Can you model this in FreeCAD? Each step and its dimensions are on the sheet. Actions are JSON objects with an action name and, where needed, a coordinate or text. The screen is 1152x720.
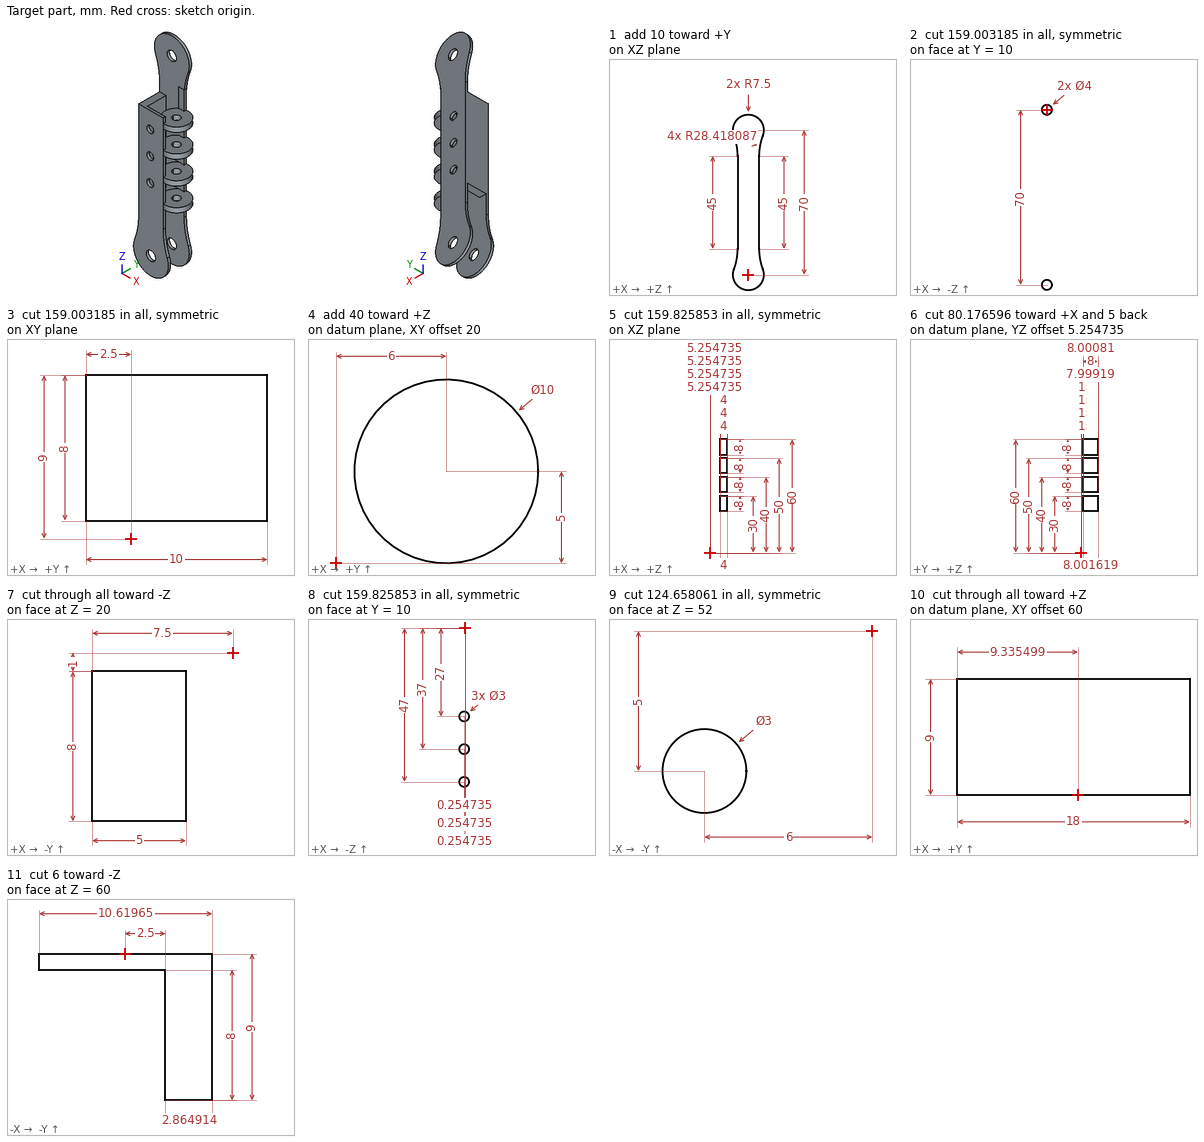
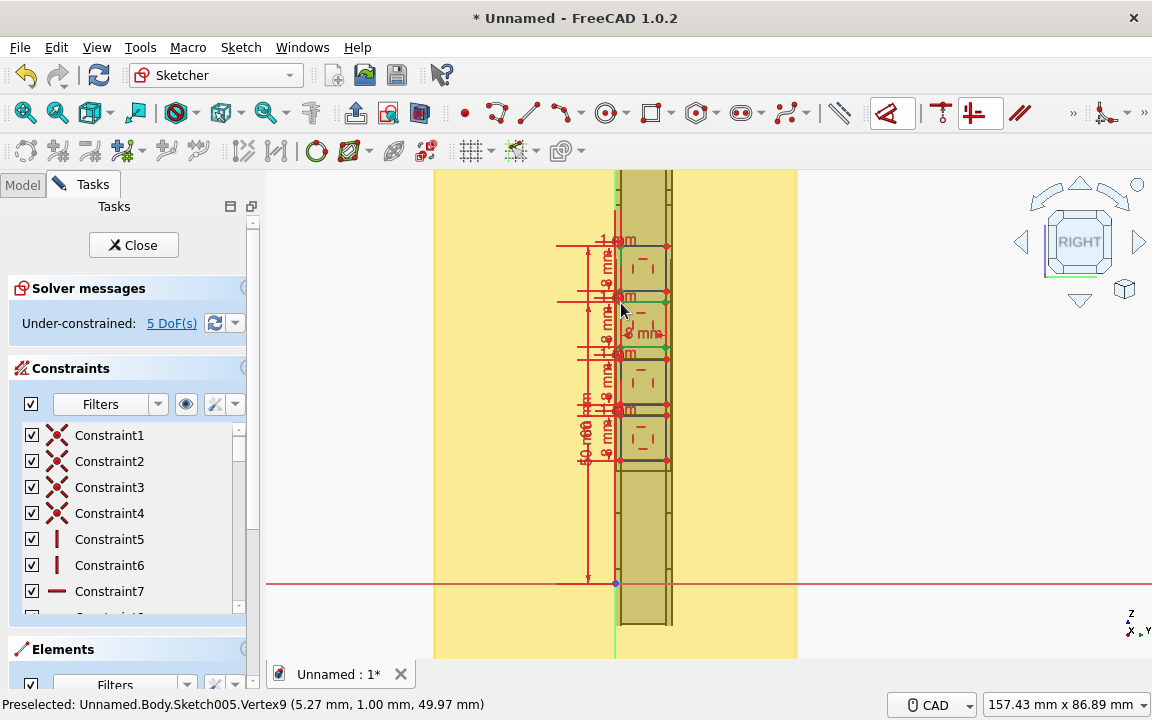
{"action": "left_click", "coordinate": [621, 360]}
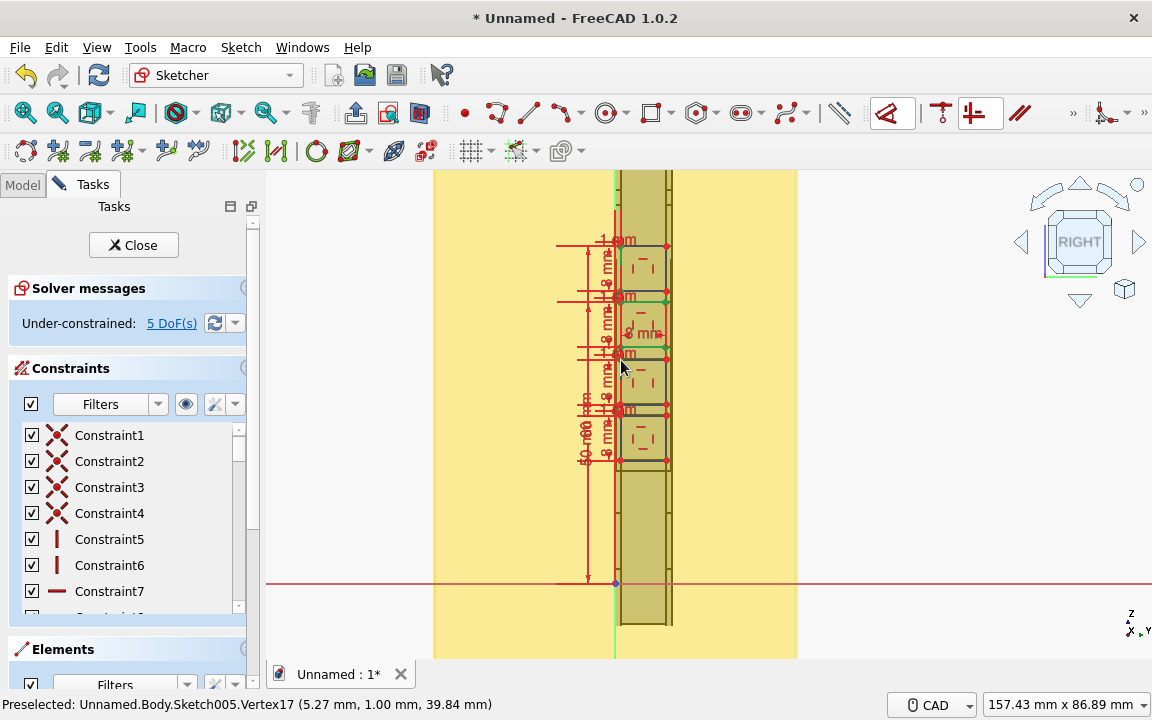
{"action": "left_click", "coordinate": [910, 114]}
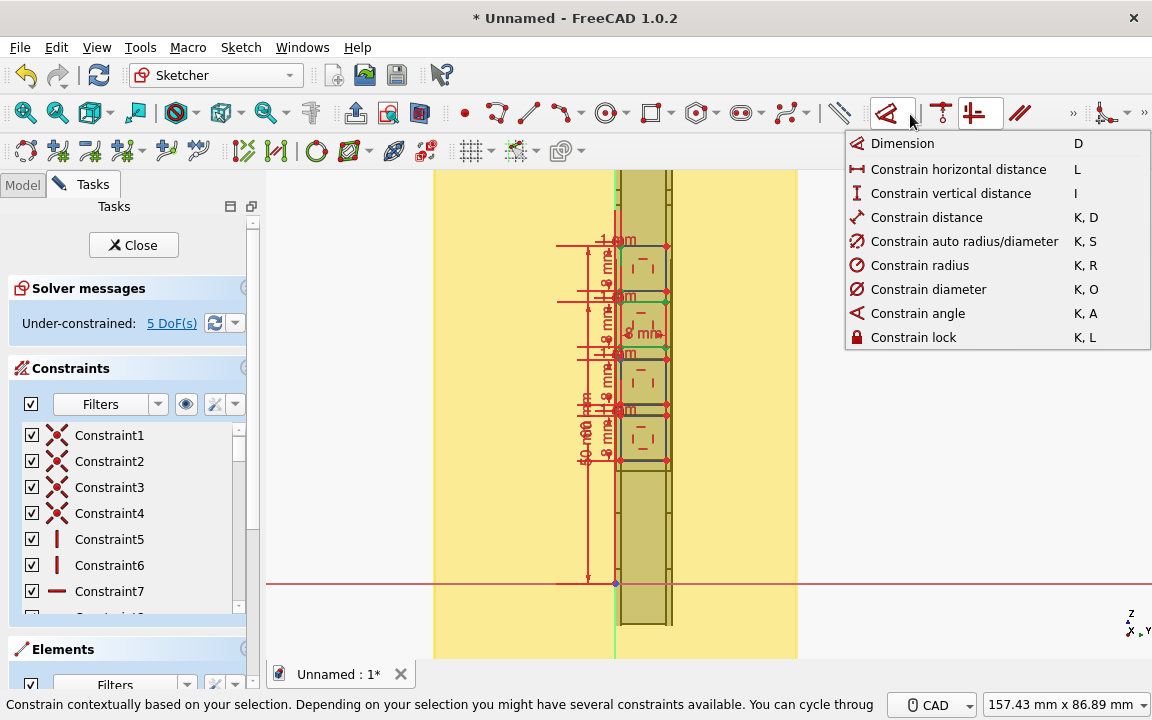
{"action": "left_click", "coordinate": [998, 193]}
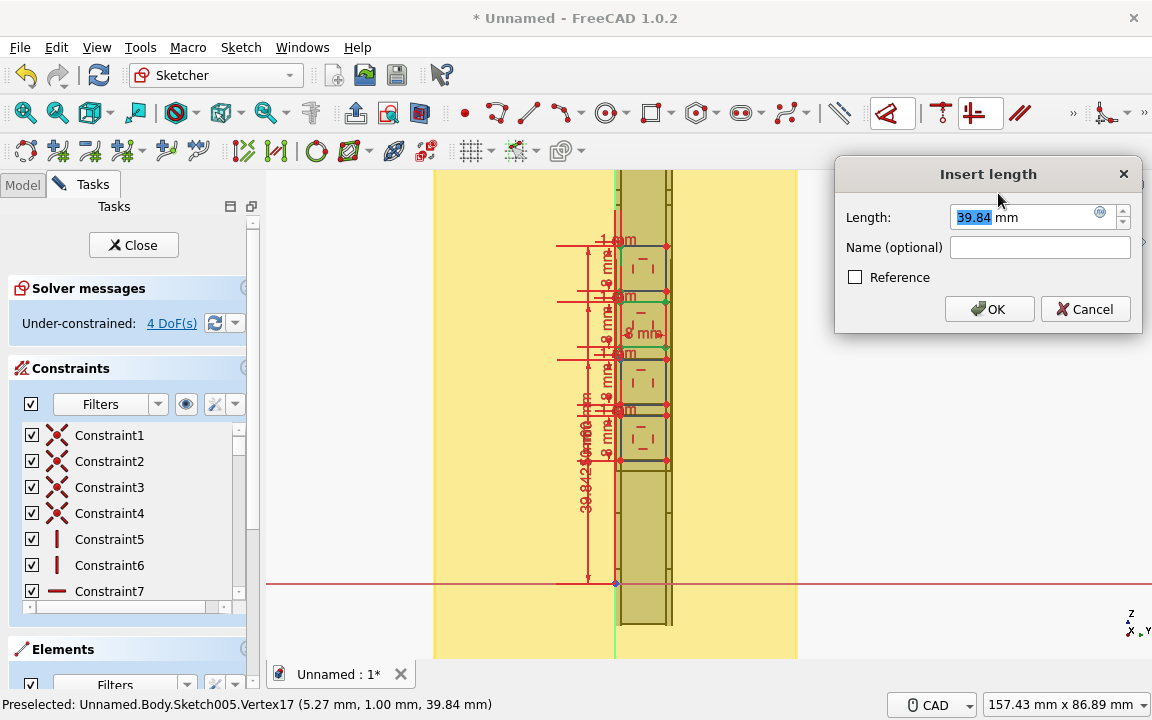
{"action": "type", "text": "40"}
{"action": "key", "text": "Return"}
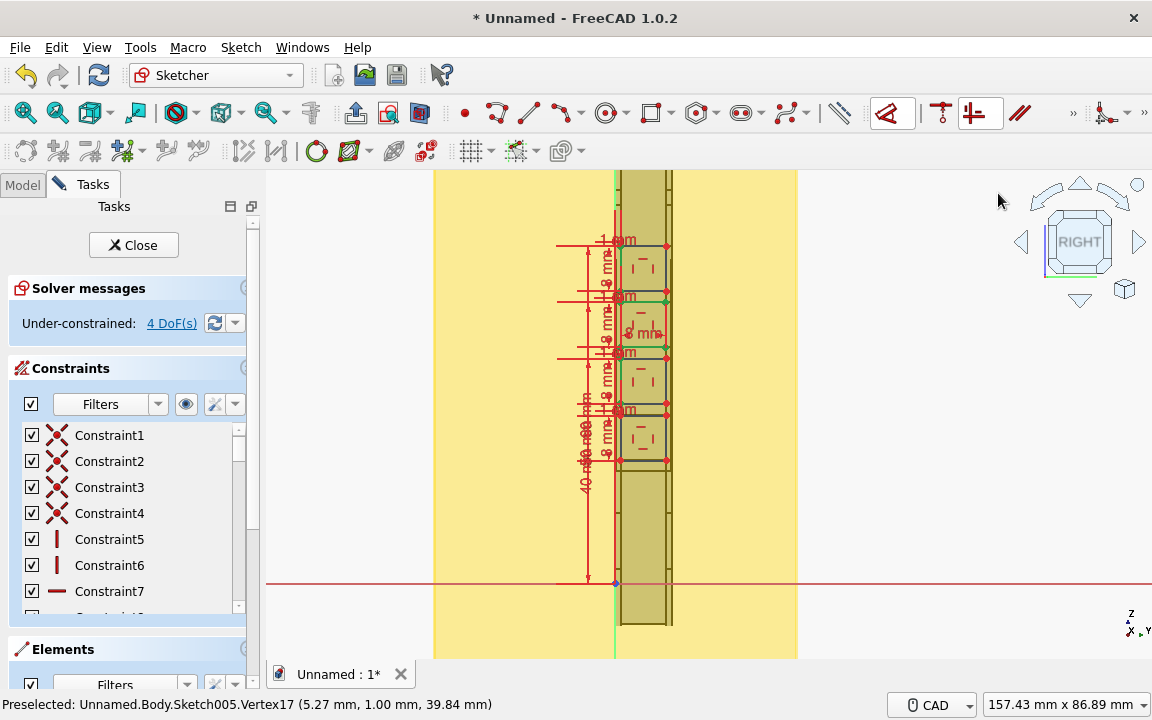
{"action": "left_click", "coordinate": [621, 416]}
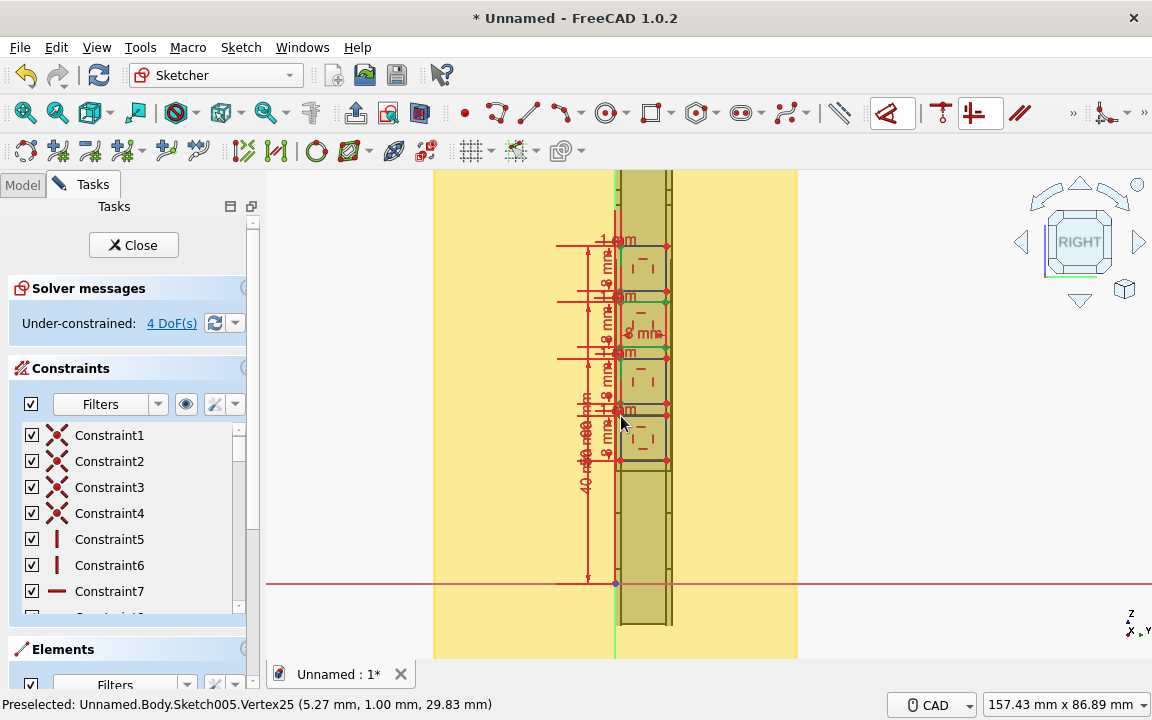
{"action": "left_click", "coordinate": [910, 114]}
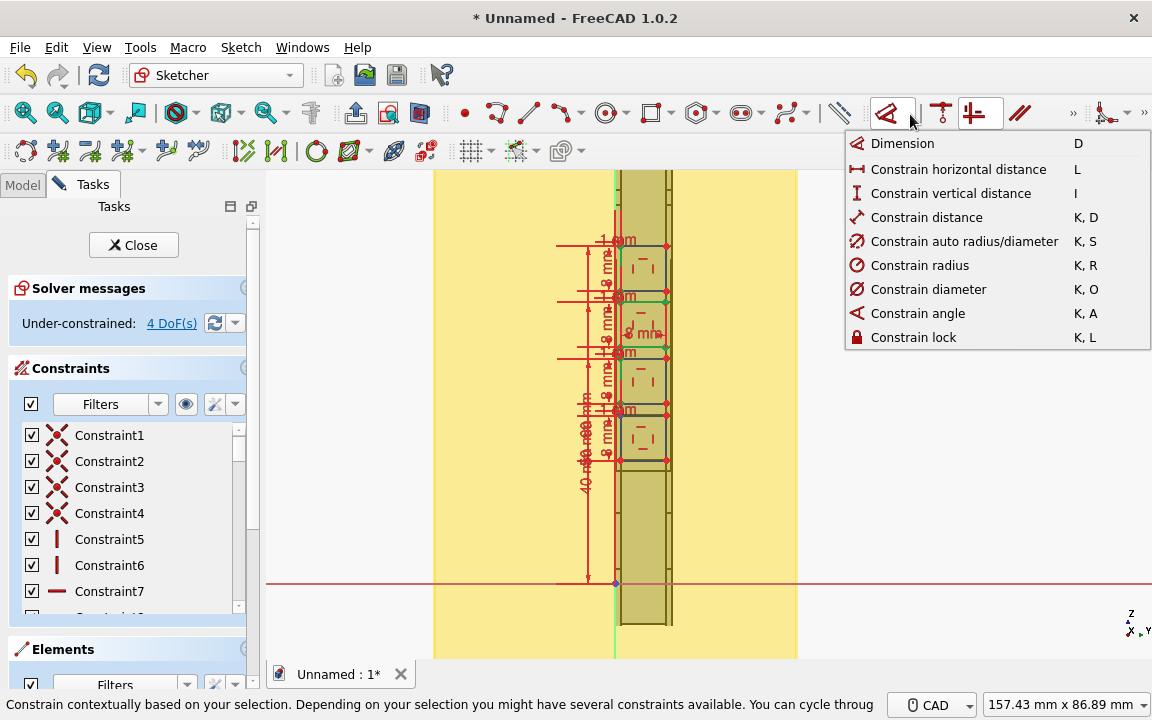
{"action": "left_click", "coordinate": [998, 193]}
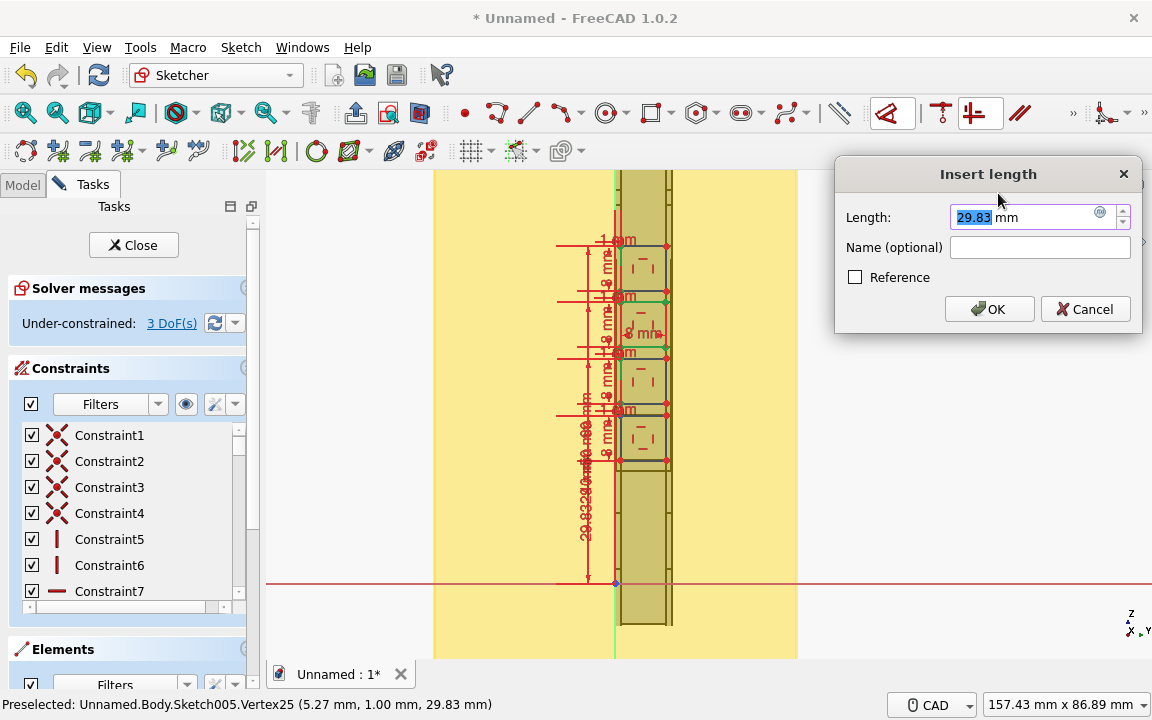
{"action": "type", "text": "30"}
{"action": "key", "text": "Return"}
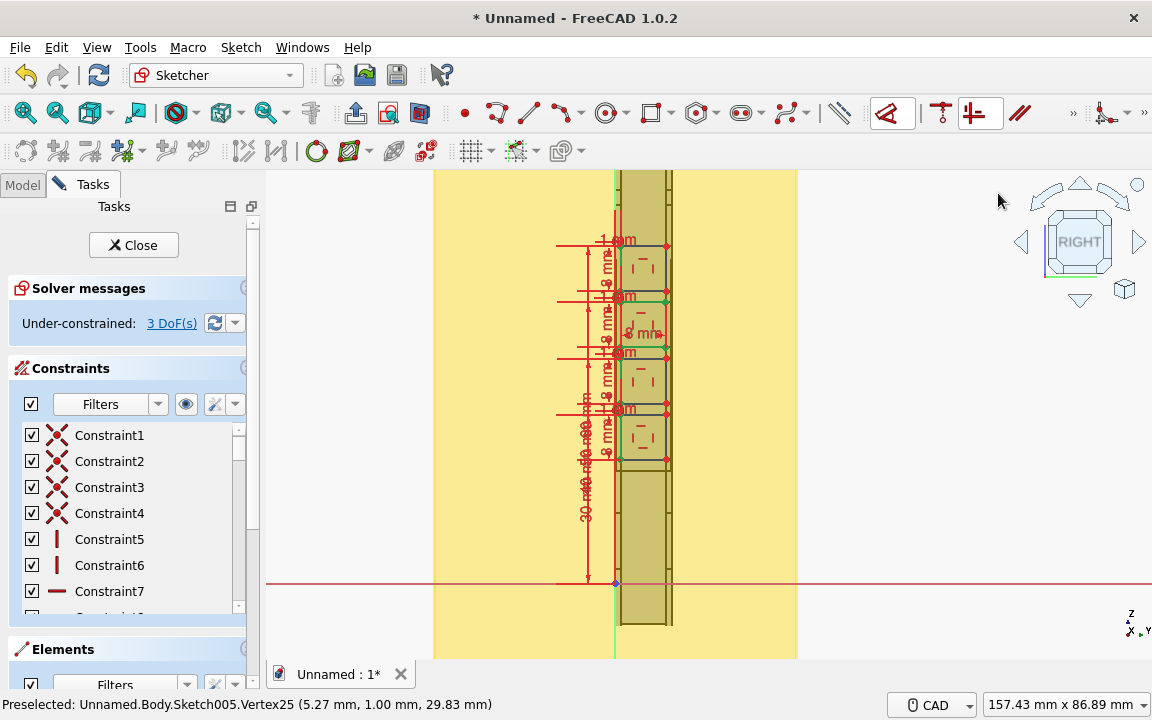
{"action": "scroll", "coordinate": [634, 291], "scroll_direction": "up", "scroll_amount": 2}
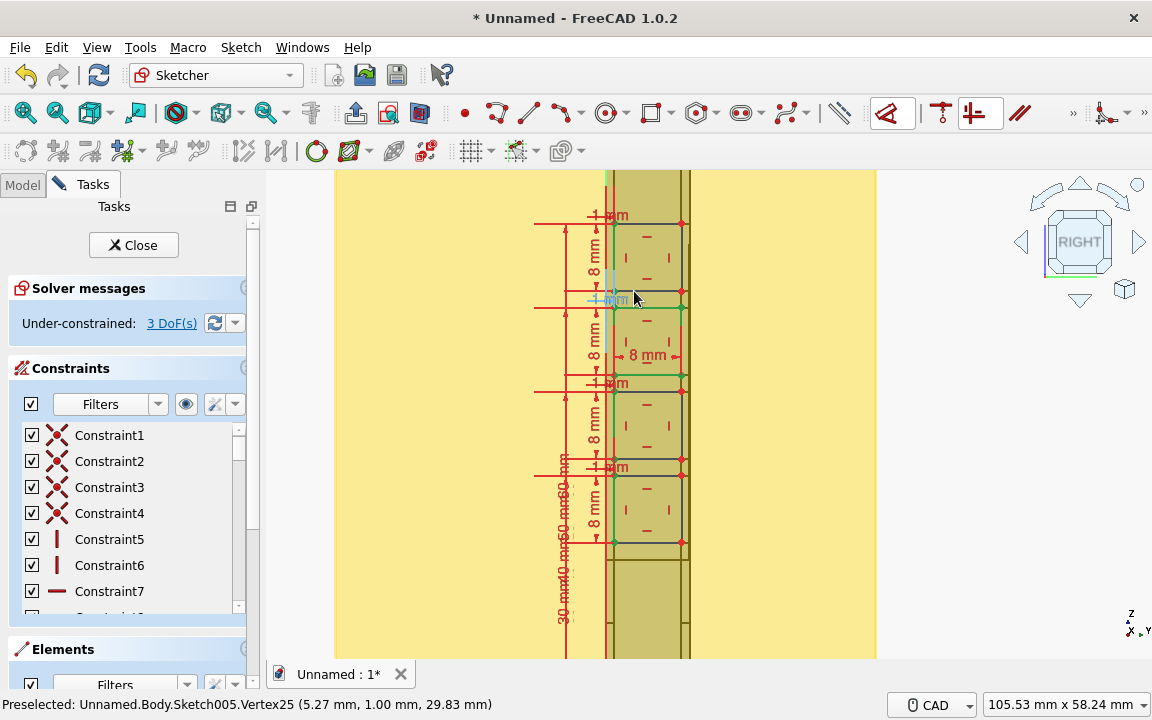
{"action": "left_click", "coordinate": [634, 291]}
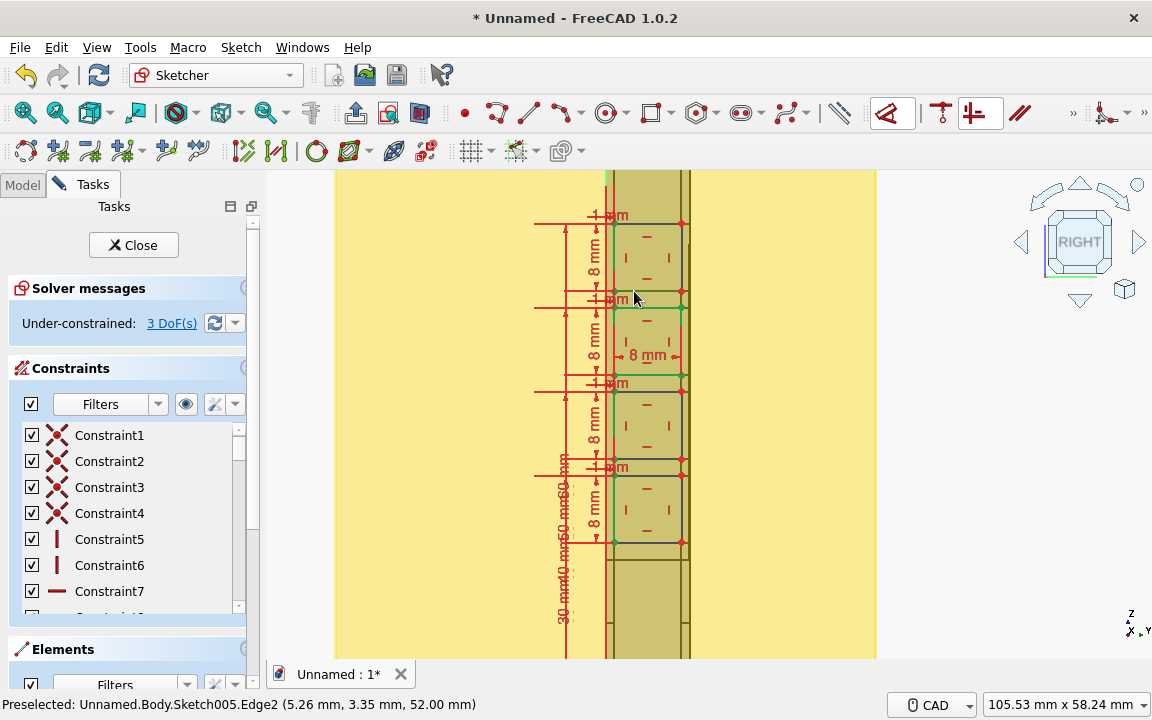
{"action": "key", "text": "l"}